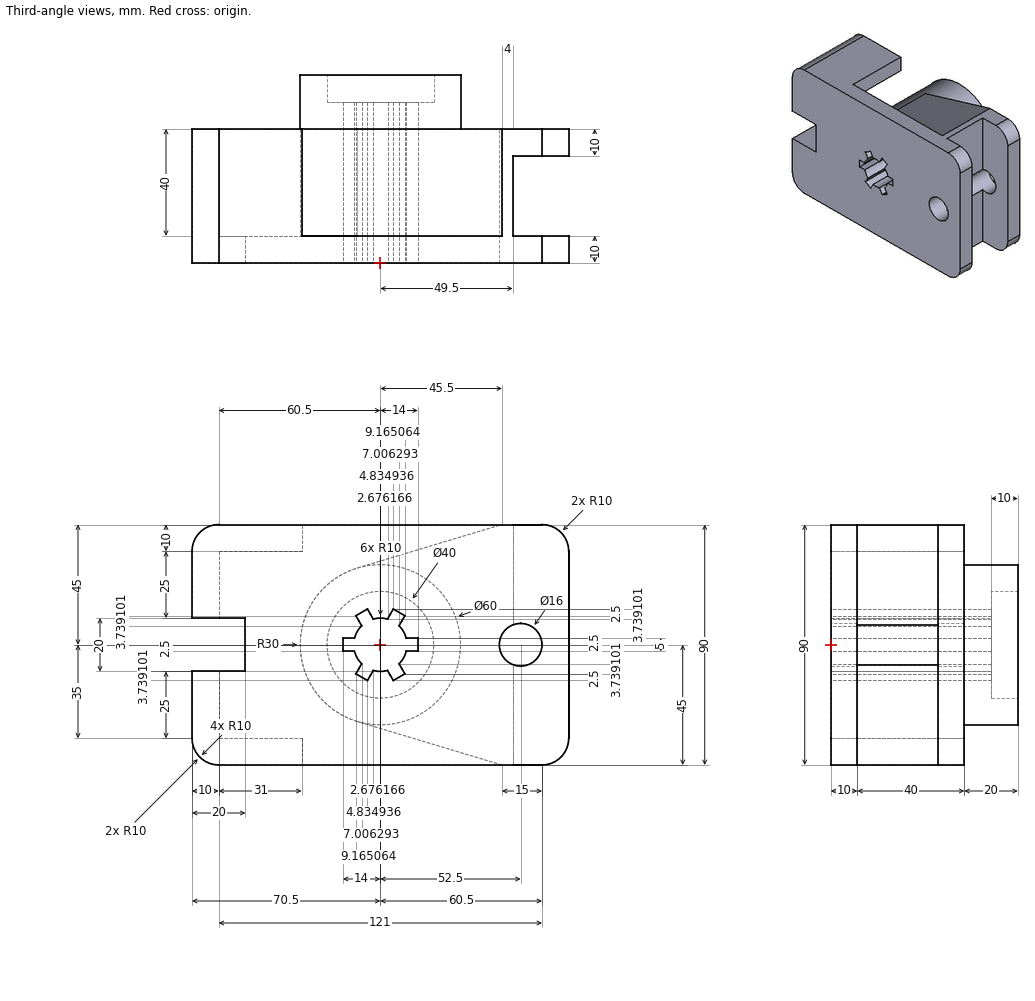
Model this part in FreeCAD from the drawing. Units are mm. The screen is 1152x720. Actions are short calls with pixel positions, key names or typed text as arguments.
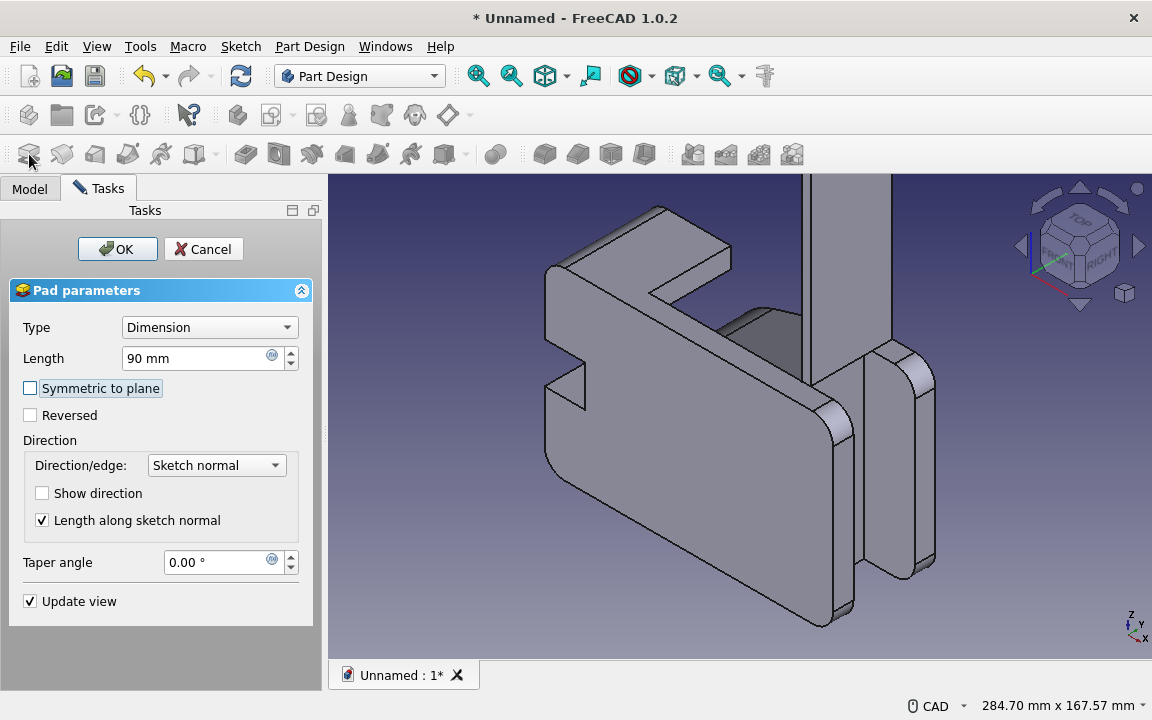
click(31, 415)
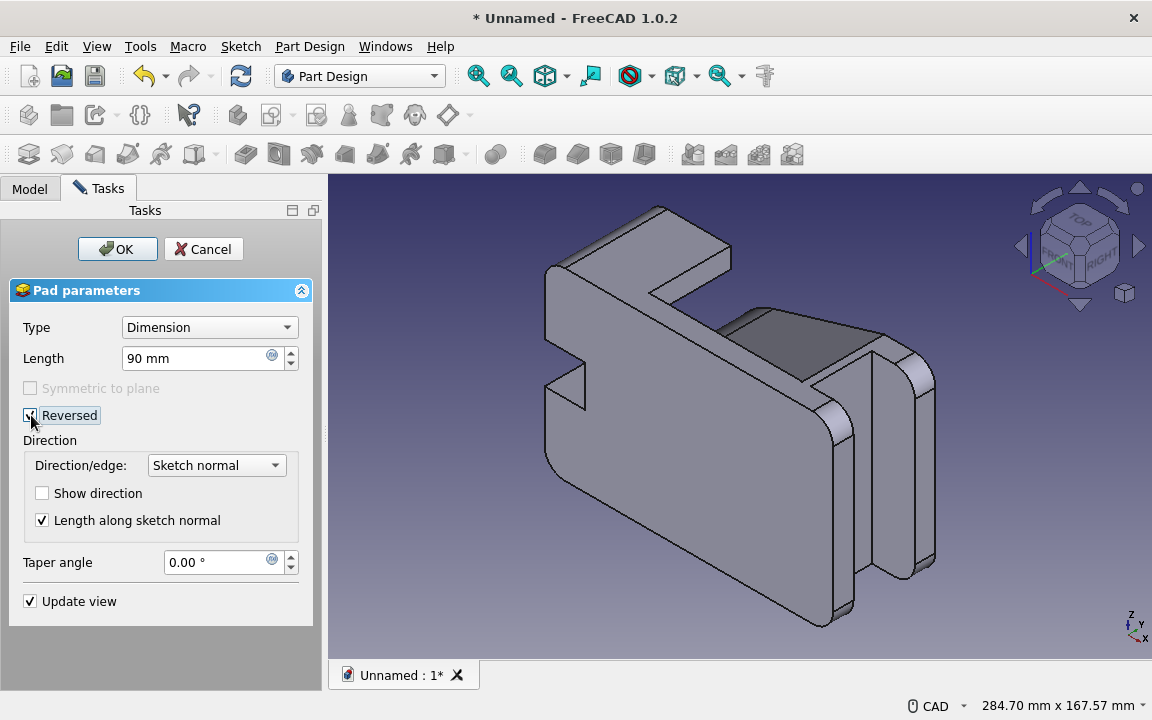
click(118, 249)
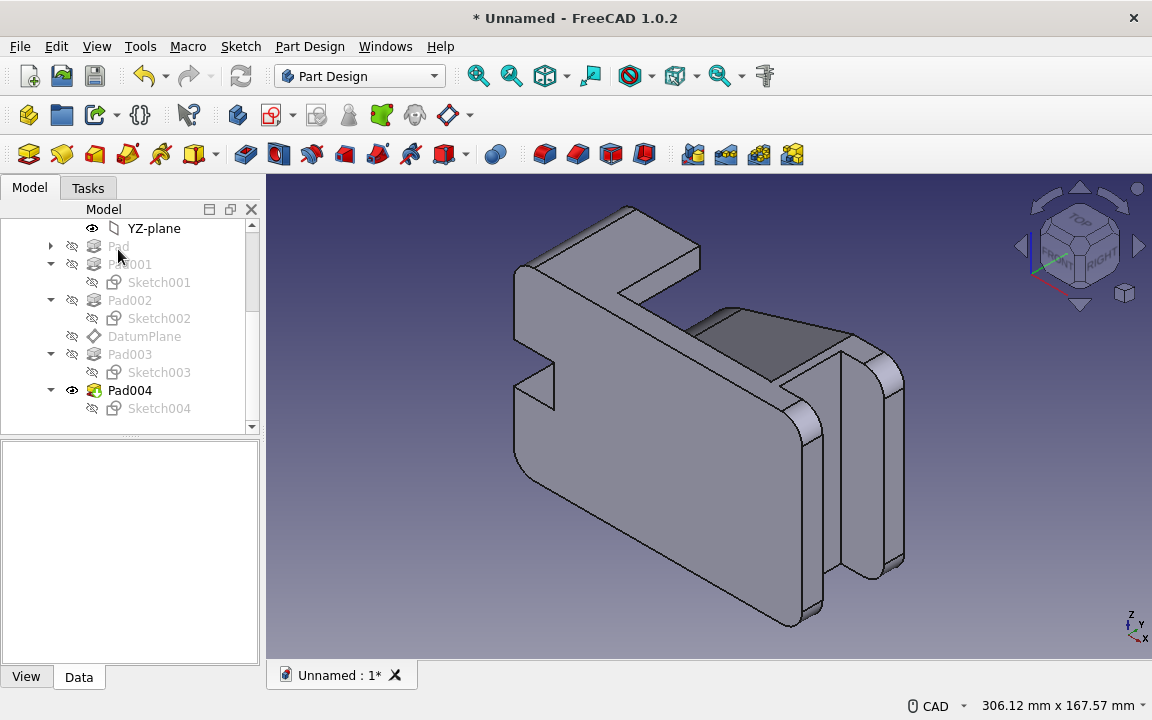
key(4)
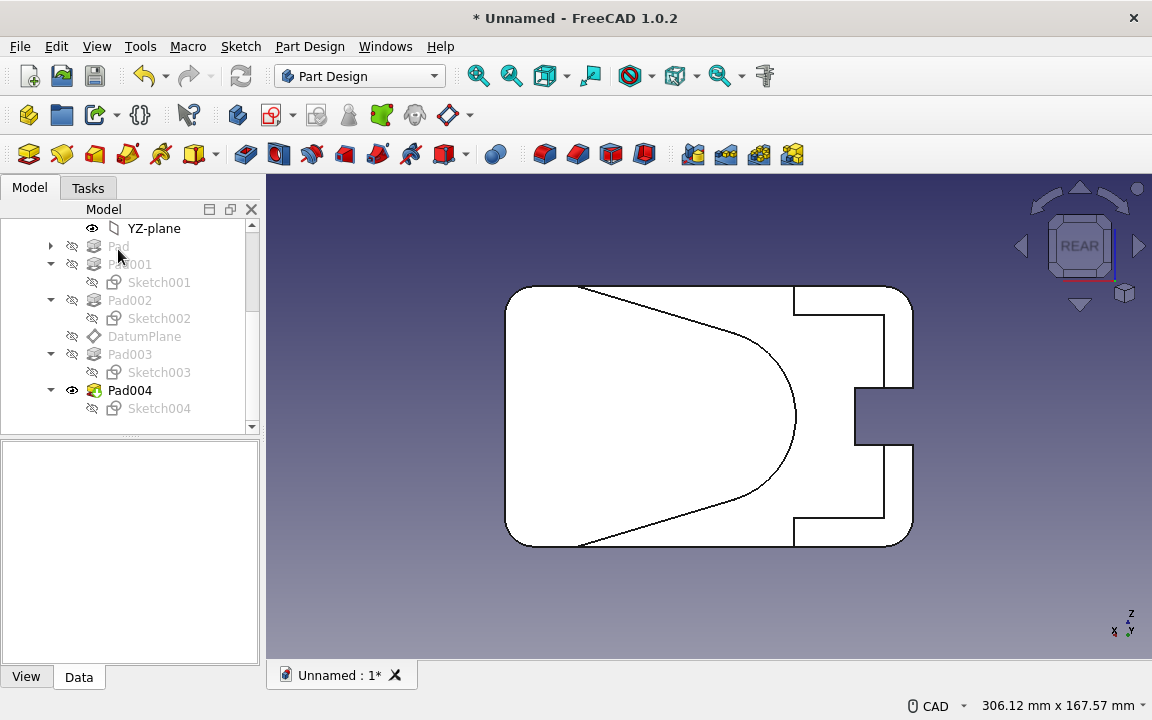
click(609, 416)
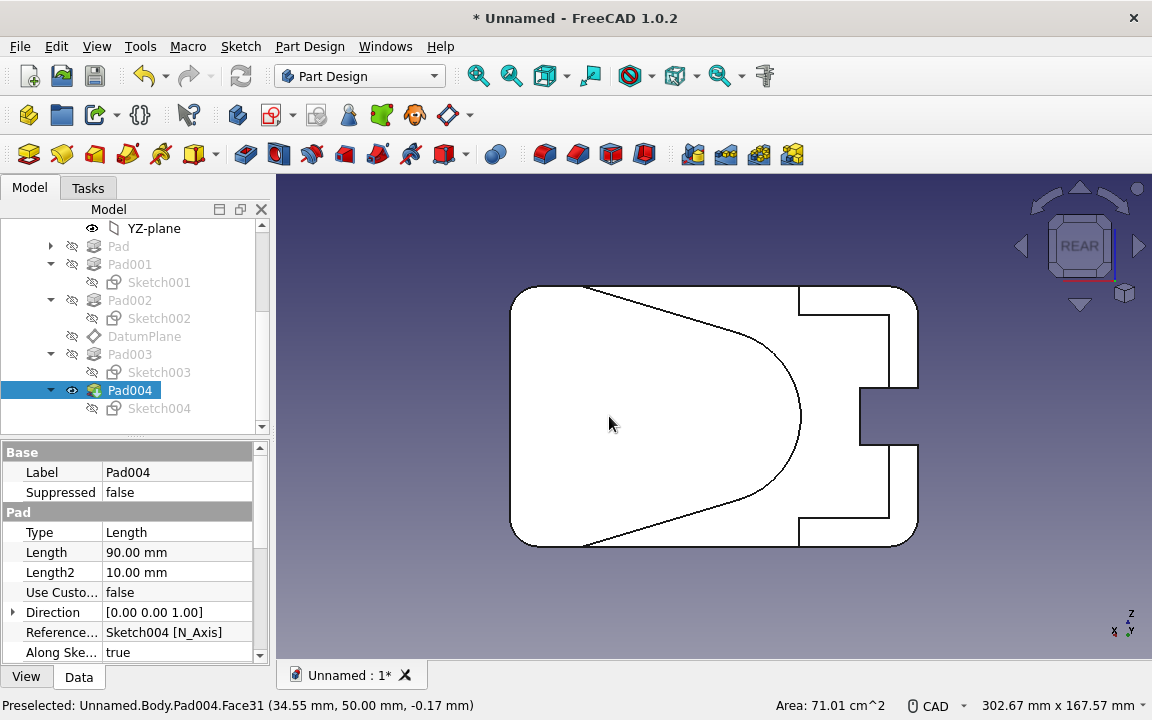
click(270, 116)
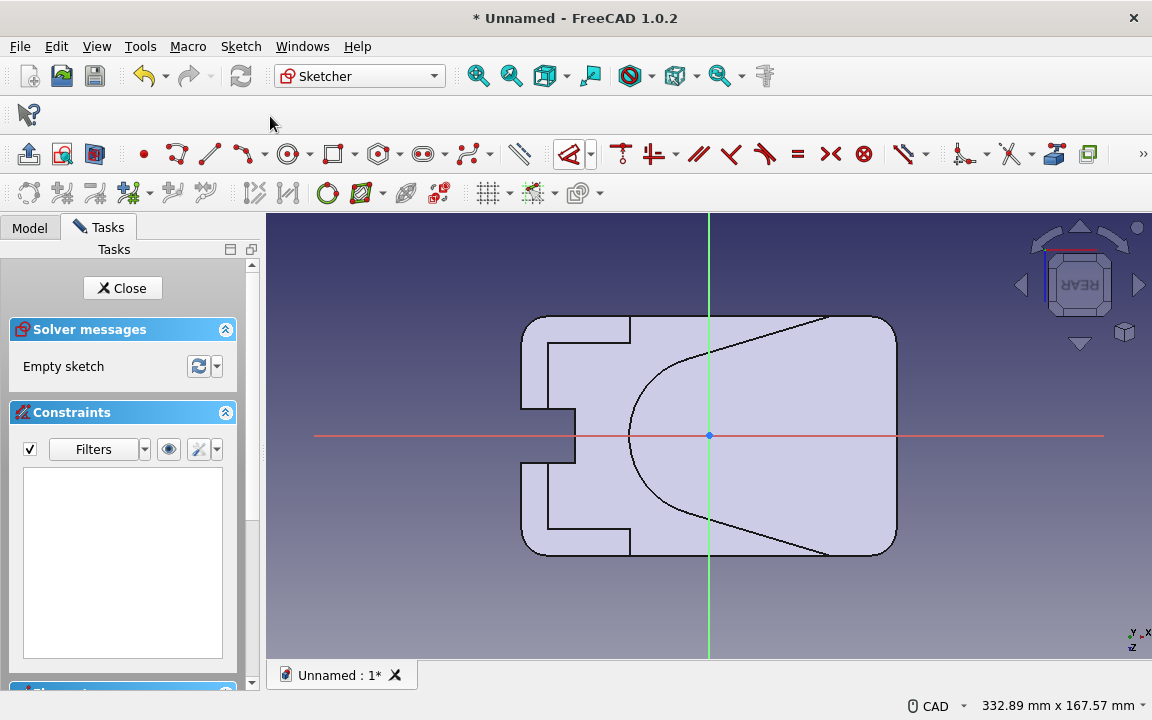
scroll(890, 436, up, 9)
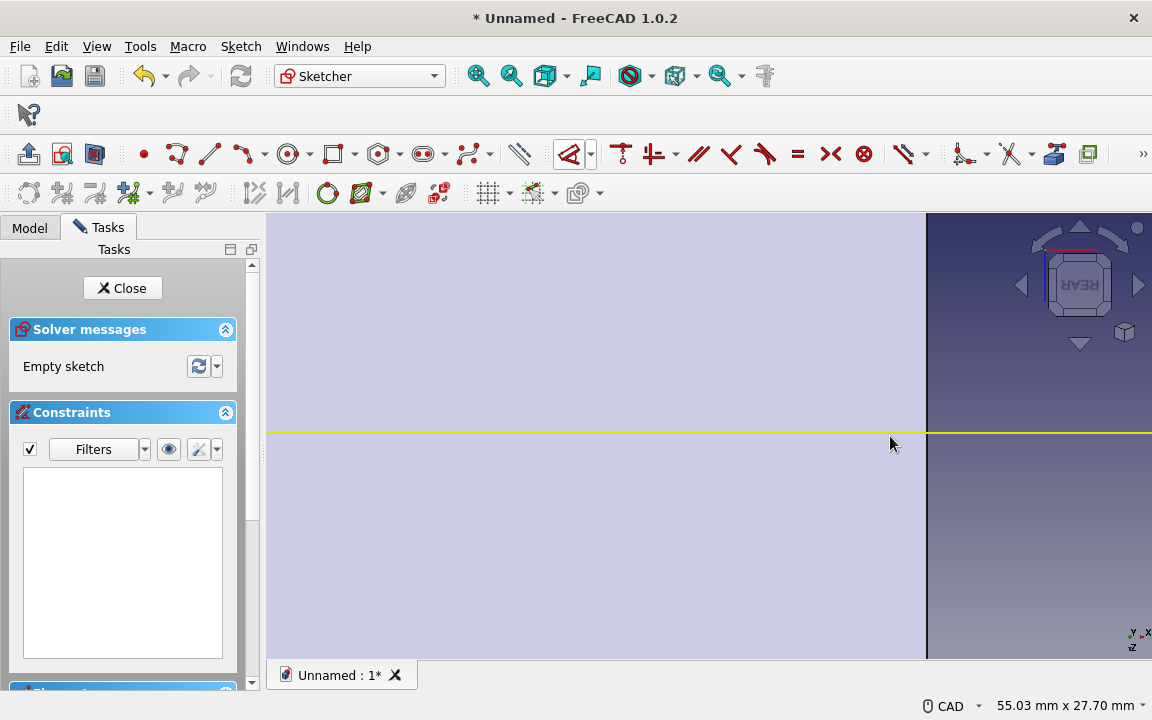
click(288, 154)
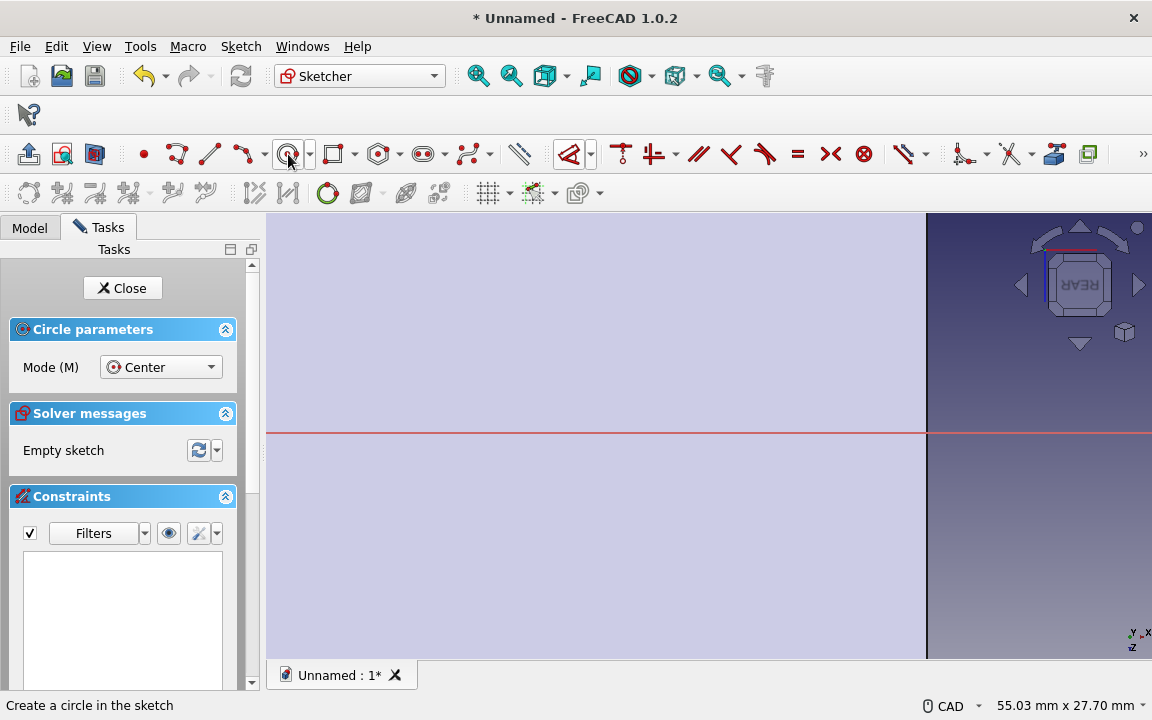
click(637, 433)
move(728, 342)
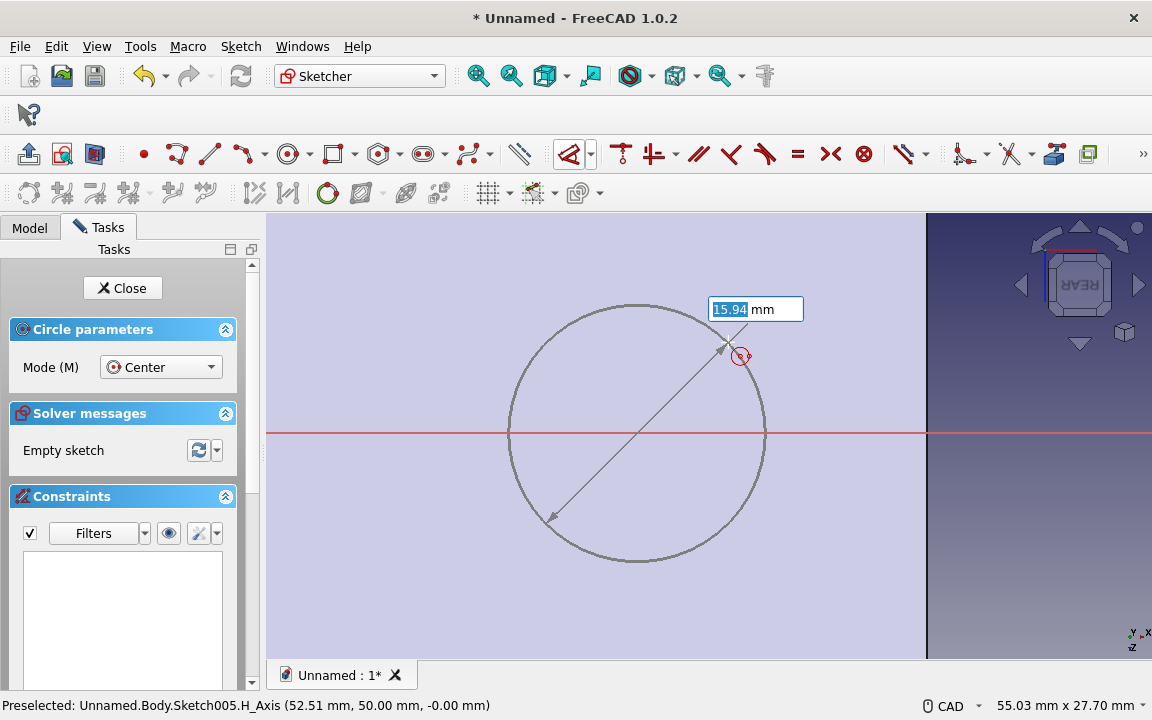
text(16)
key(Return)
key(Escape)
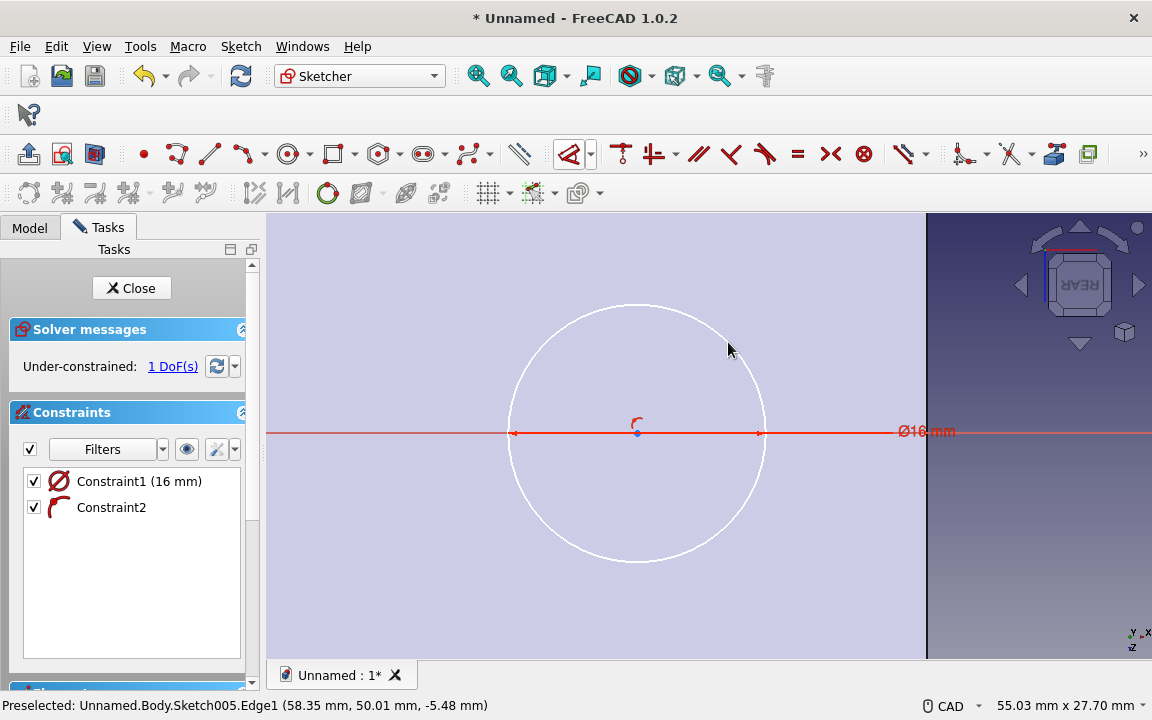
click(637, 433)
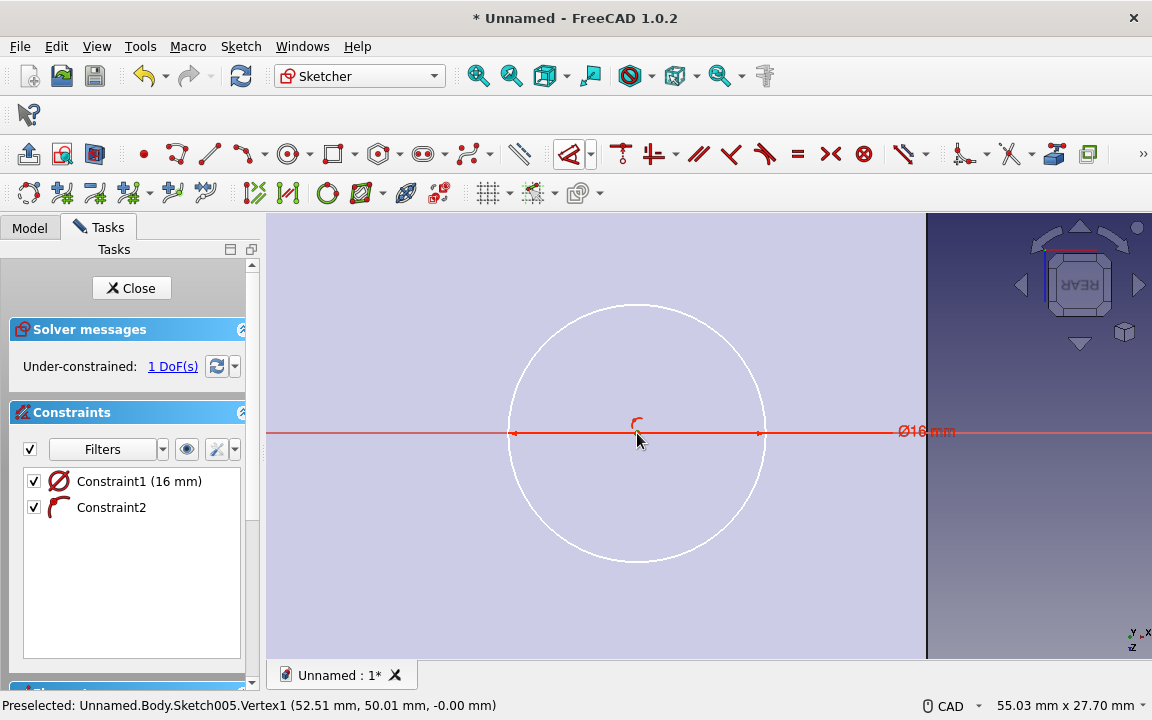
click(590, 154)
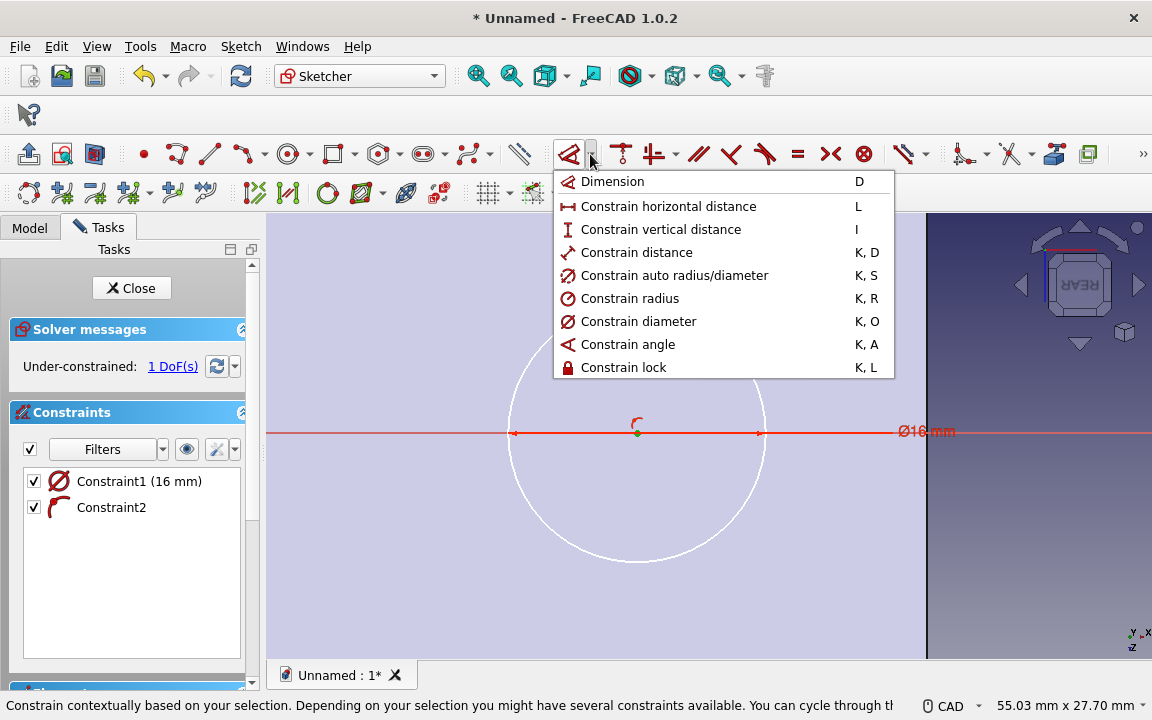
click(724, 206)